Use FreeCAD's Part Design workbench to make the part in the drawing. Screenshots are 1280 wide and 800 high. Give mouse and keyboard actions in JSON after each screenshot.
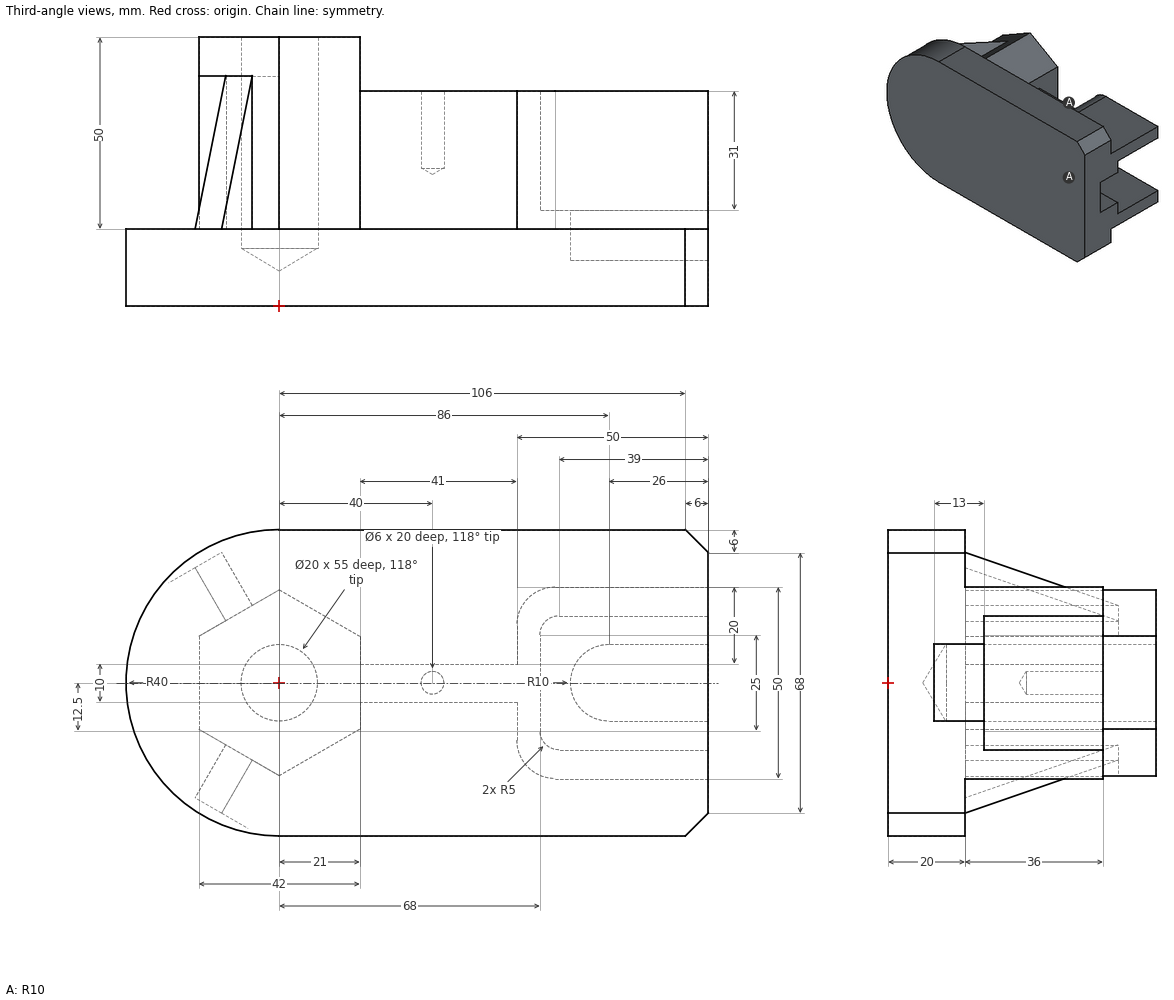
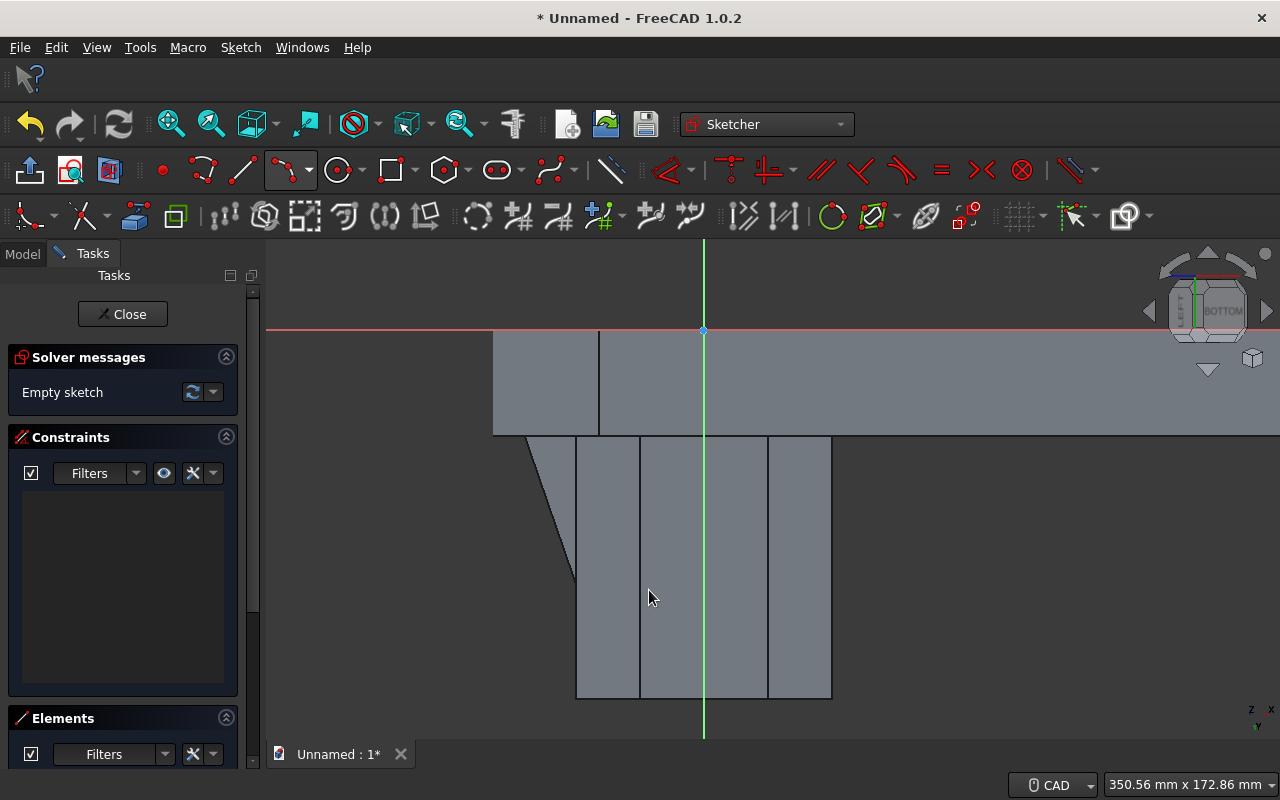
{"action": "left_click", "coordinate": [392, 170]}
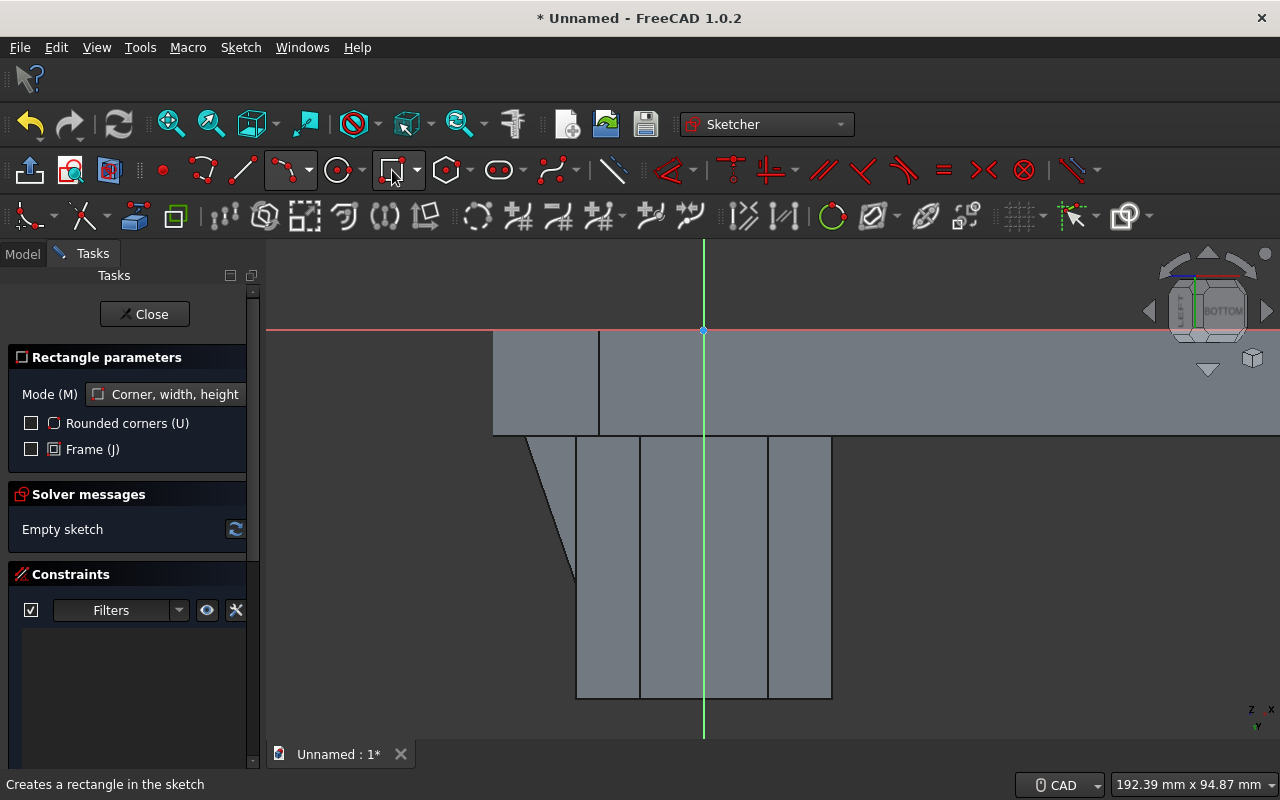
{"action": "left_click", "coordinate": [683, 436]}
{"action": "mouse_move", "coordinate": [725, 646]}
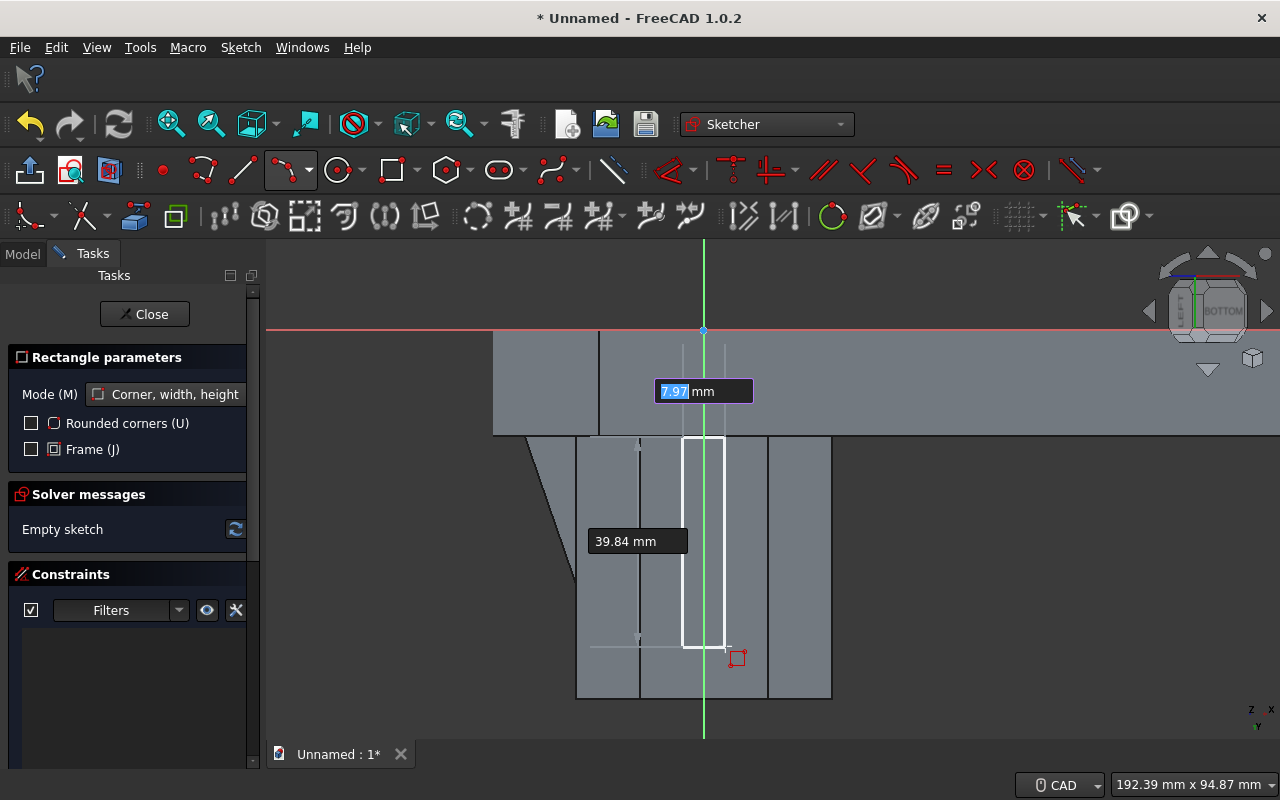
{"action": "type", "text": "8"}
{"action": "key", "text": "Tab"}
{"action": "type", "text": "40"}
{"action": "key", "text": "Return"}
{"action": "key", "text": "Escape"}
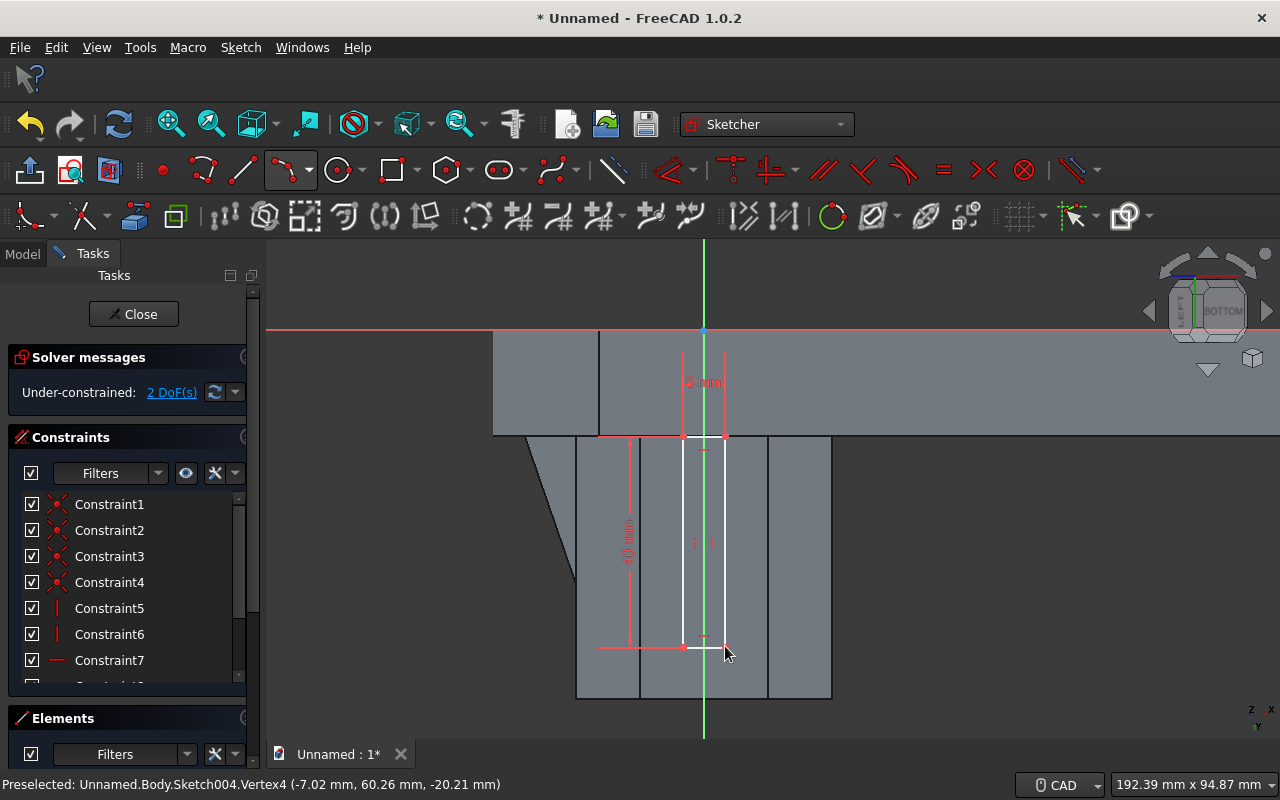
{"action": "left_click", "coordinate": [668, 170]}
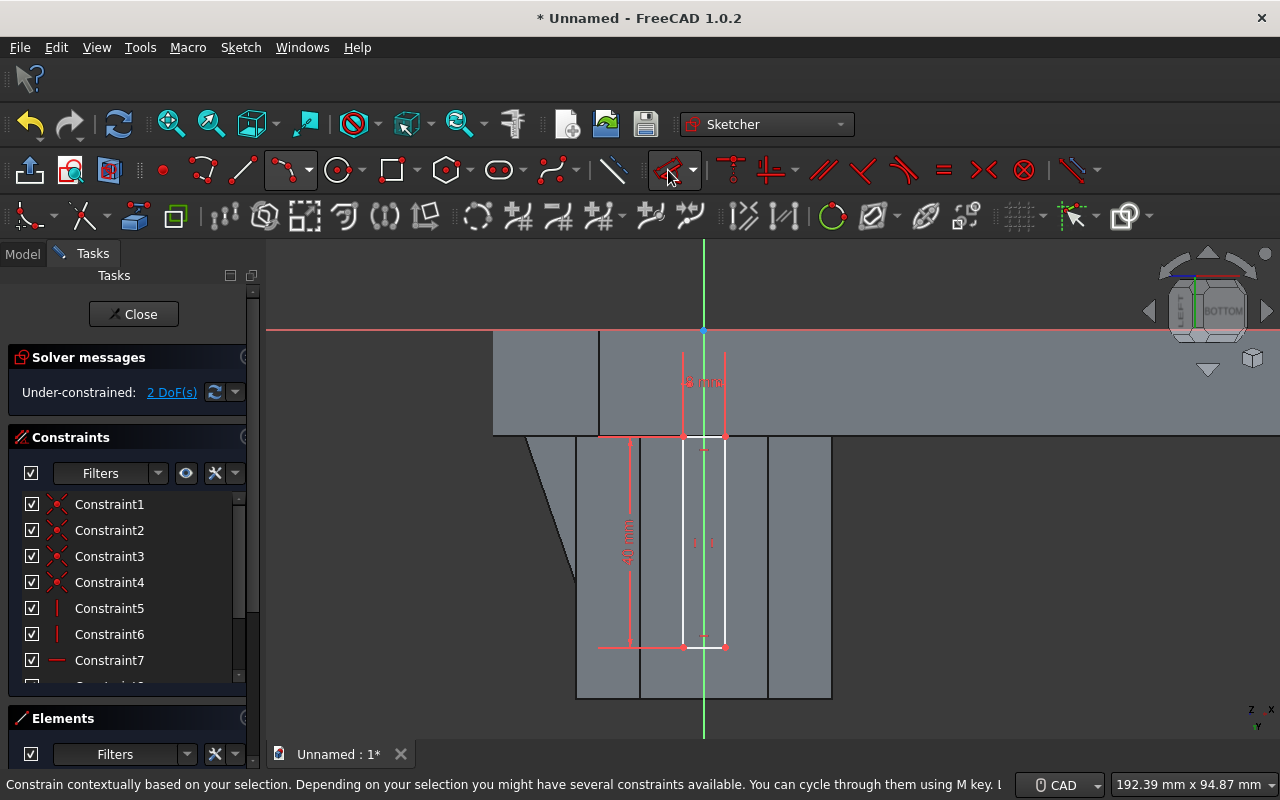
{"action": "scroll", "coordinate": [683, 437], "scroll_direction": "up", "scroll_amount": 4}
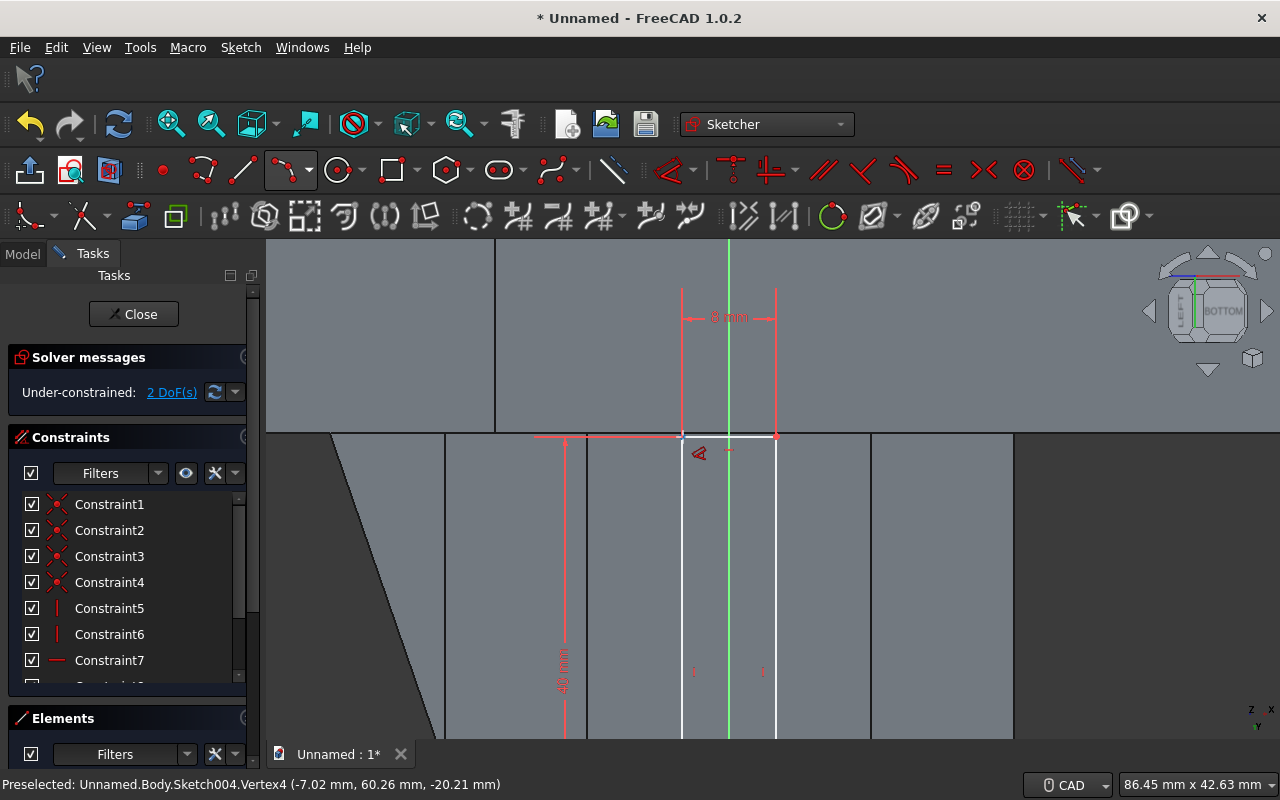
{"action": "left_click", "coordinate": [682, 437]}
{"action": "left_click", "coordinate": [706, 471]}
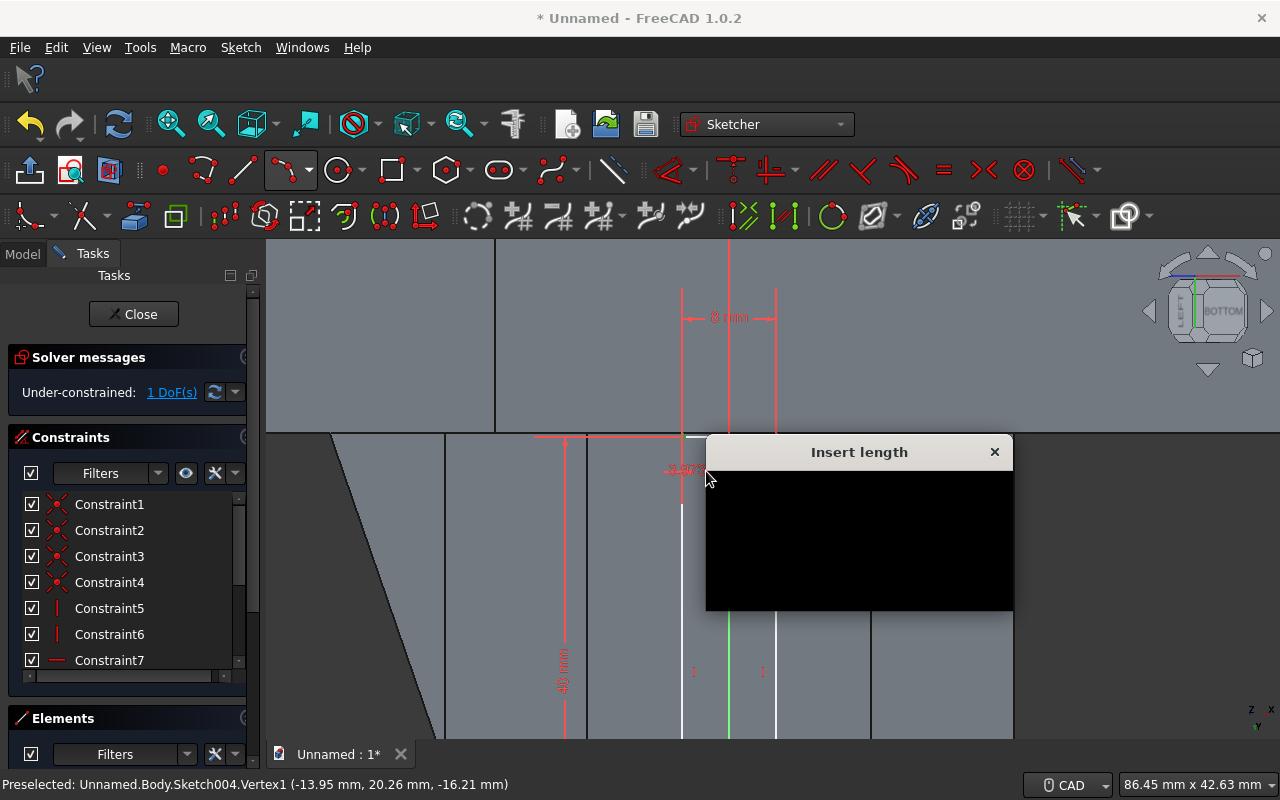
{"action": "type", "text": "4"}
{"action": "key", "text": "Return"}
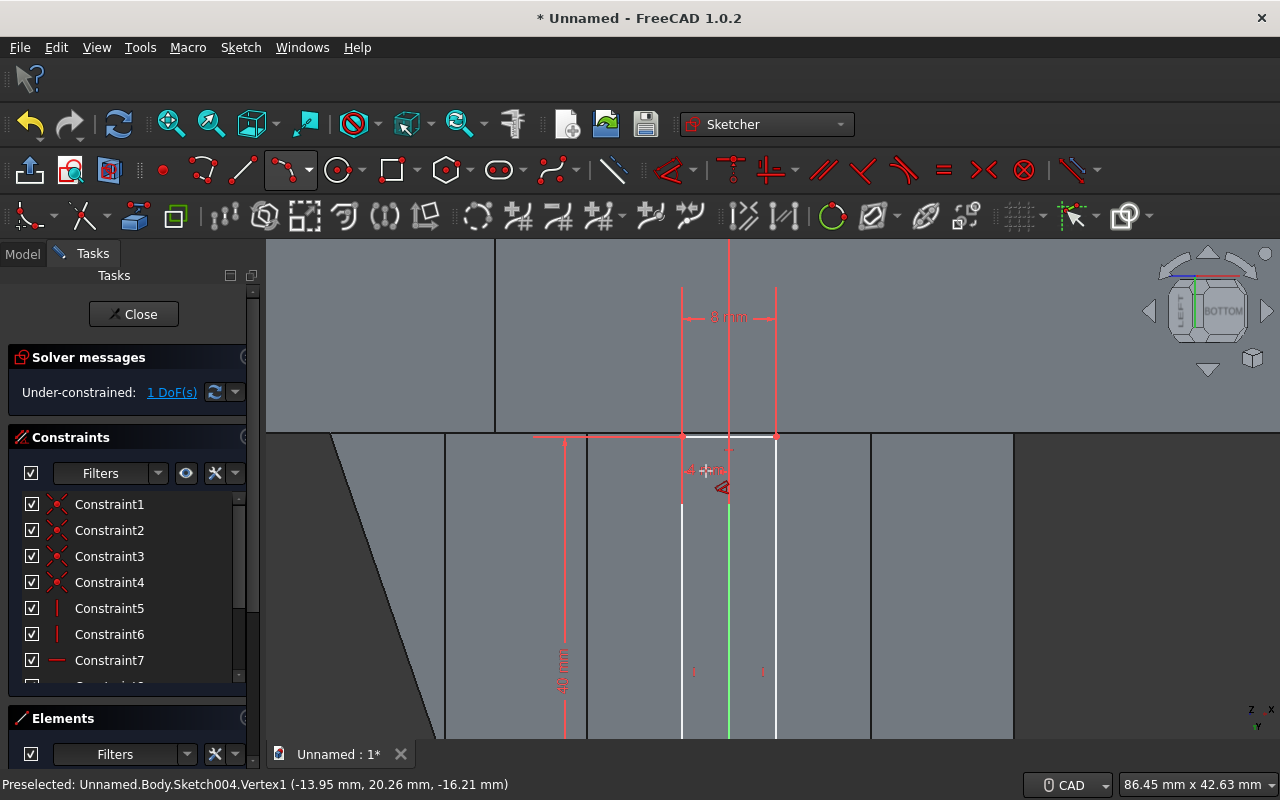
{"action": "left_click", "coordinate": [682, 437]}
{"action": "left_click", "coordinate": [648, 352]}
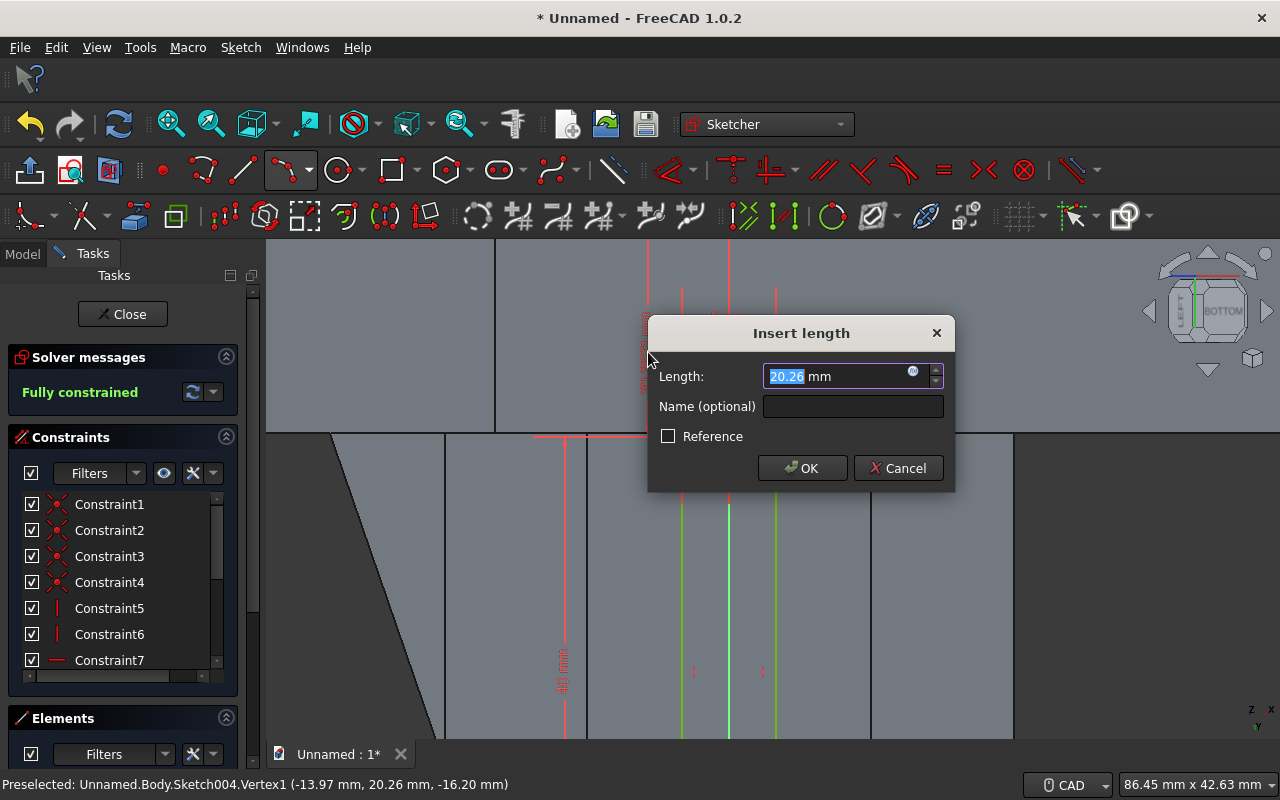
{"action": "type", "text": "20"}
{"action": "key", "text": "Return"}
{"action": "key", "text": "Escape"}